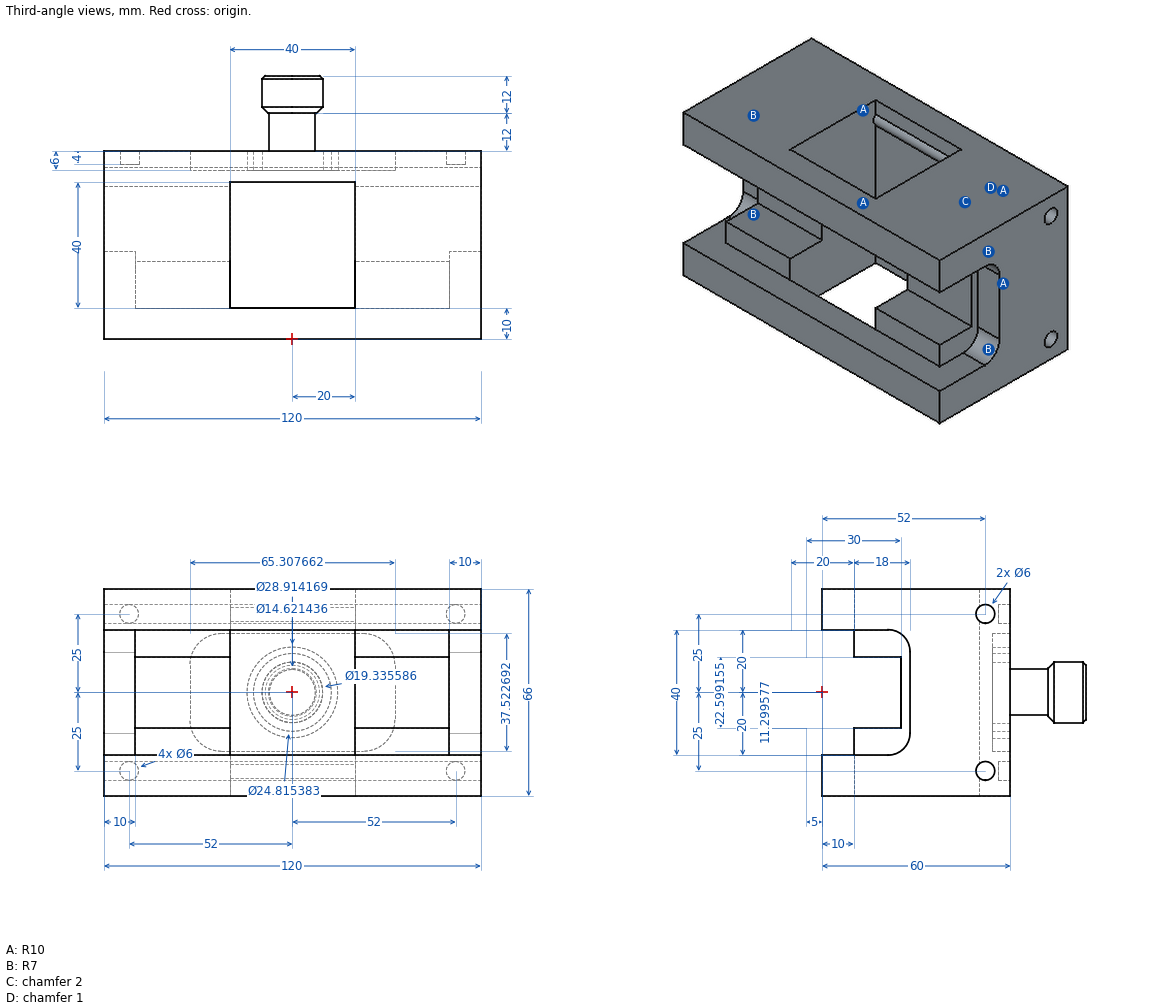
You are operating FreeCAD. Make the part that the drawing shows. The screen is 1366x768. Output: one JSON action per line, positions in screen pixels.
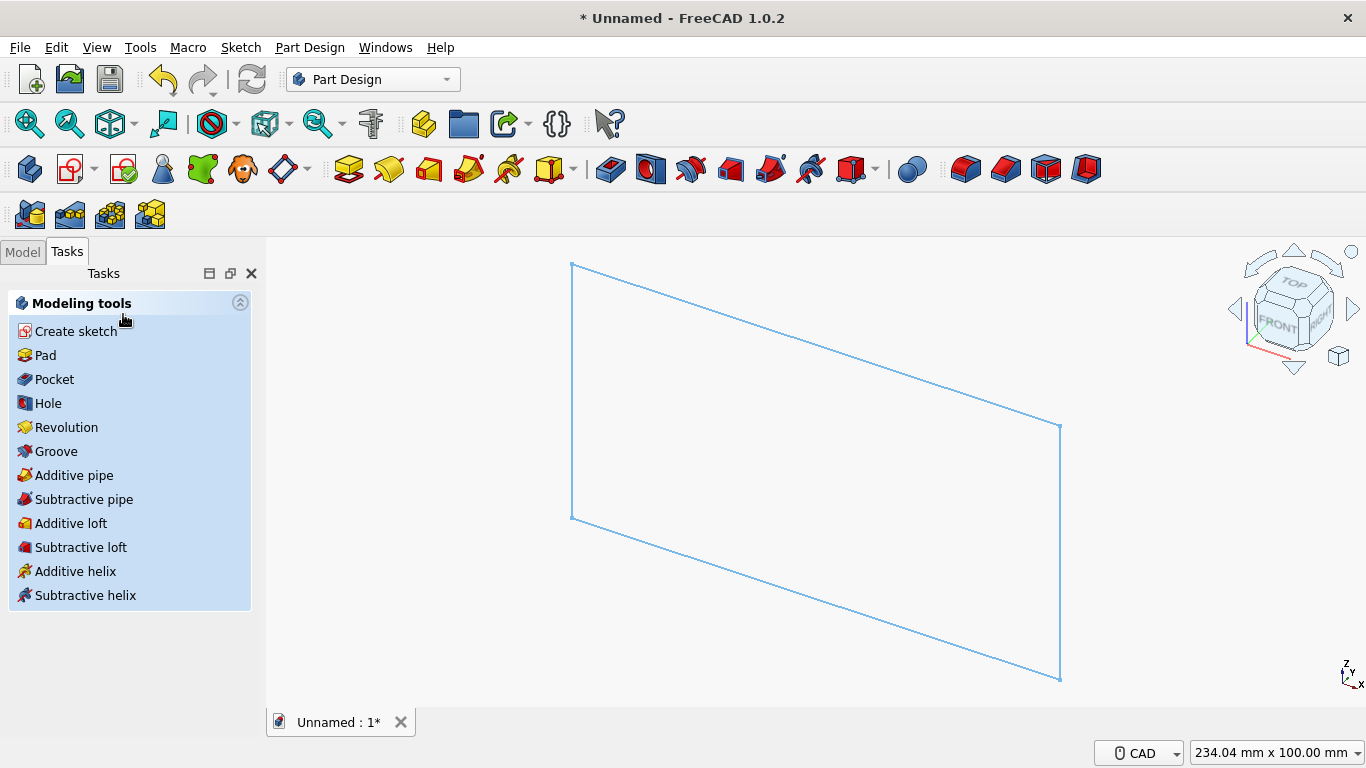
{"action": "left_click", "coordinate": [350, 170]}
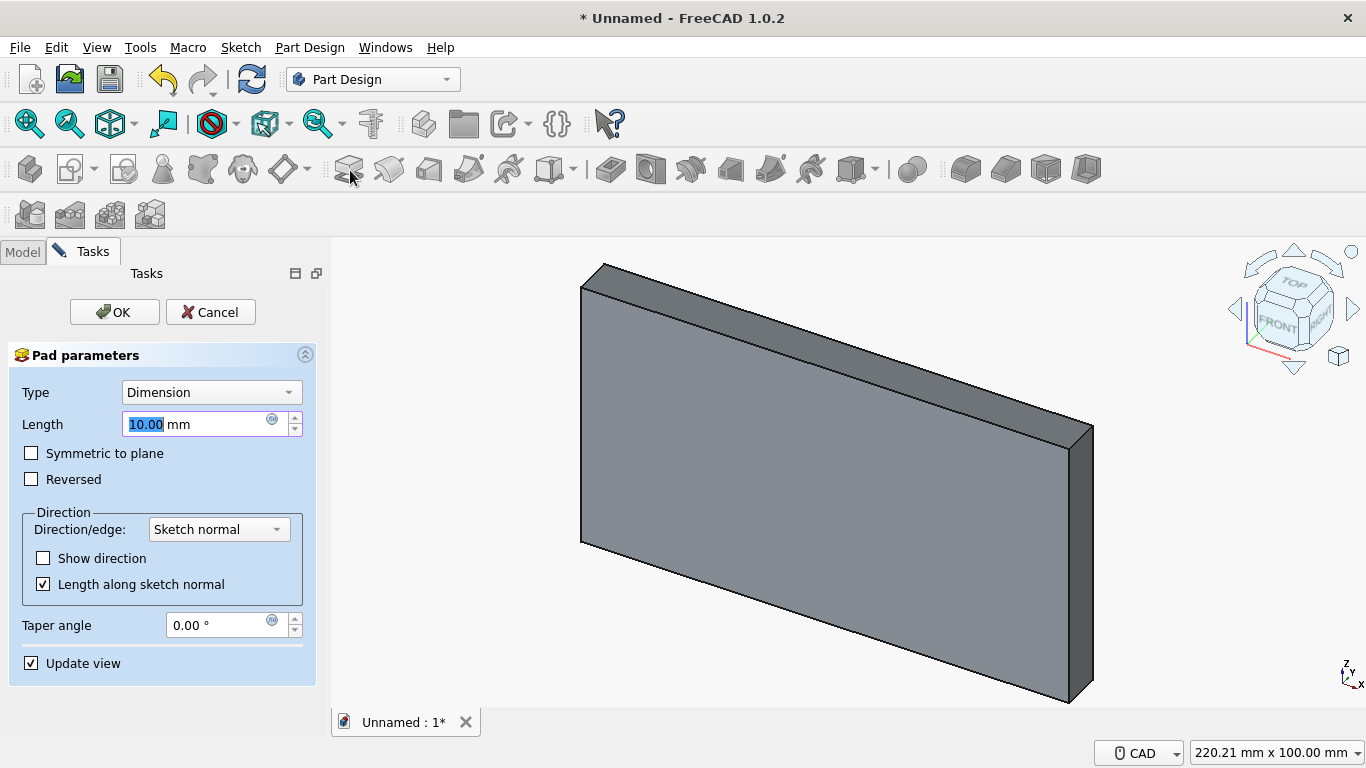
{"action": "type", "text": "60"}
{"action": "key", "text": "Tab"}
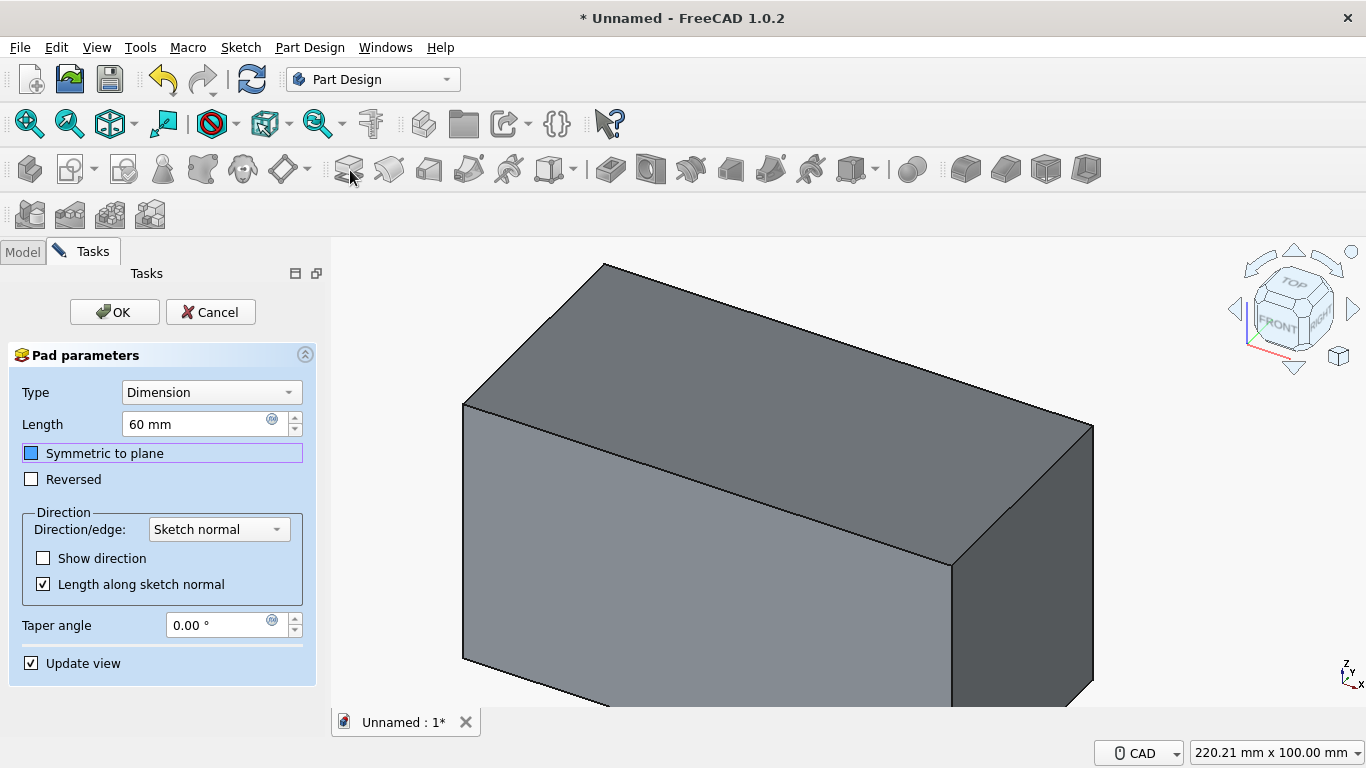
{"action": "left_click", "coordinate": [30, 479]}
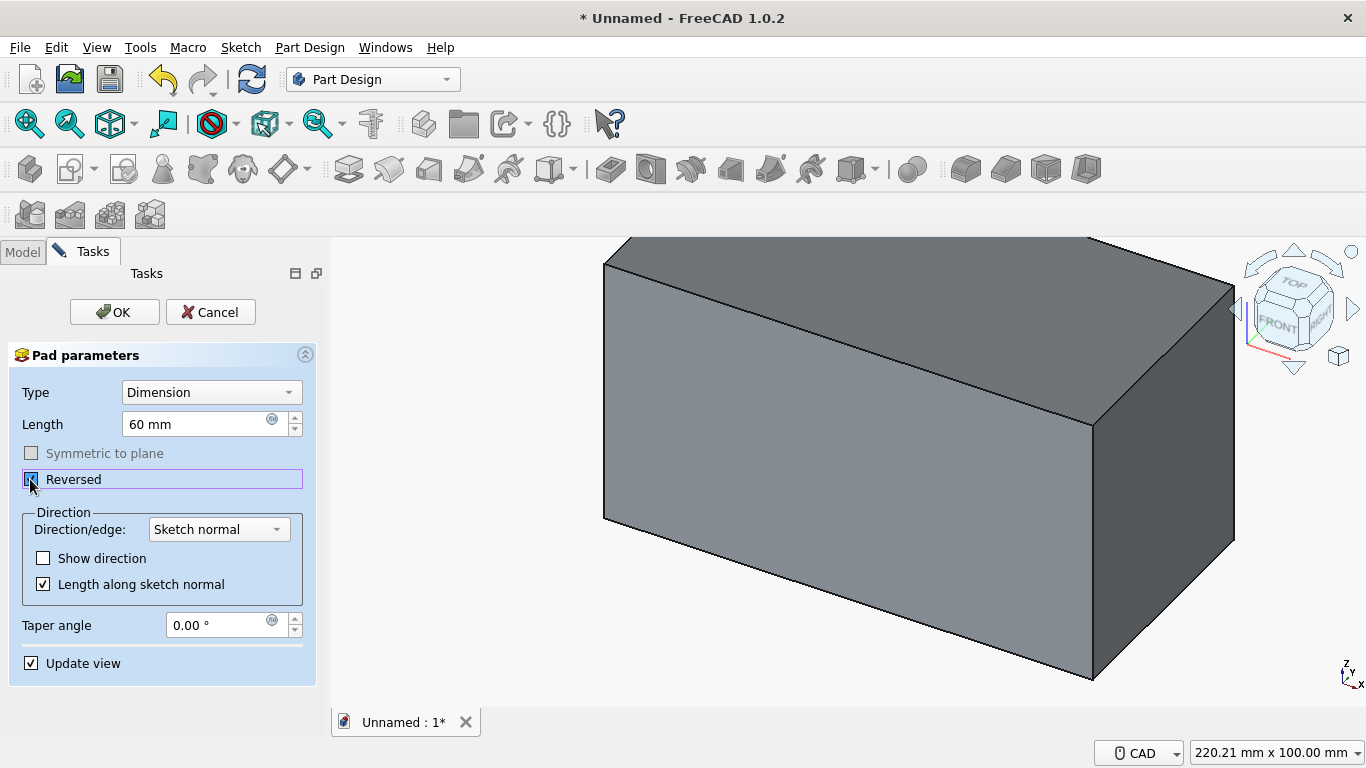
{"action": "left_click", "coordinate": [115, 312]}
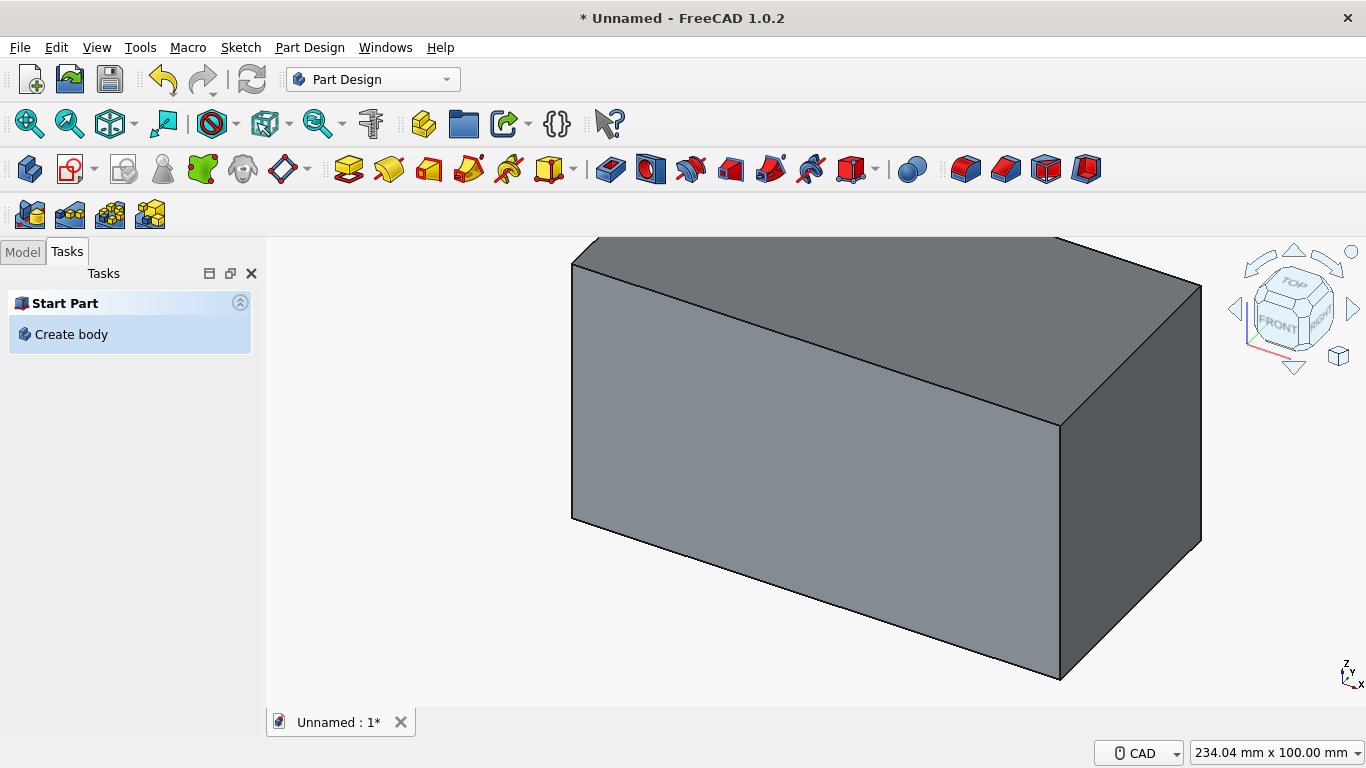
{"action": "left_click", "coordinate": [30, 124]}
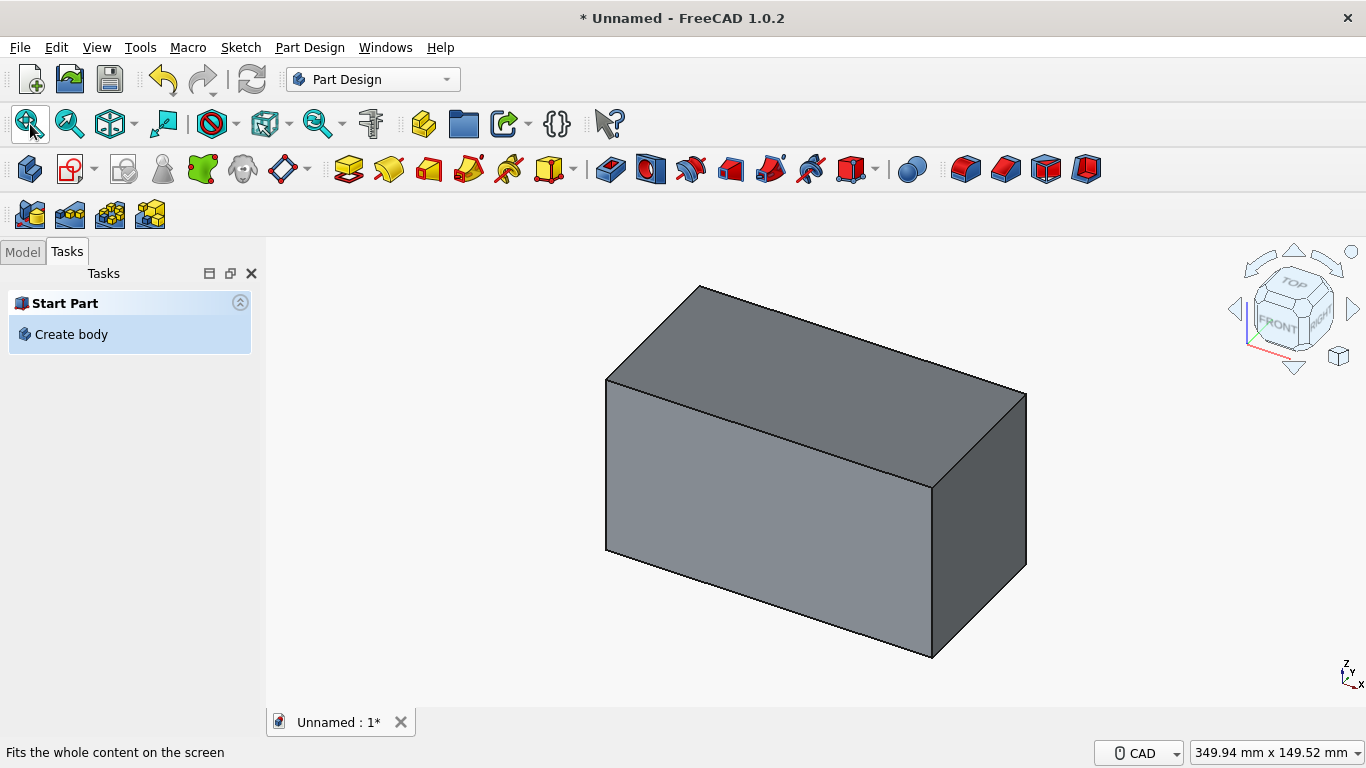
{"action": "left_click", "coordinate": [979, 525]}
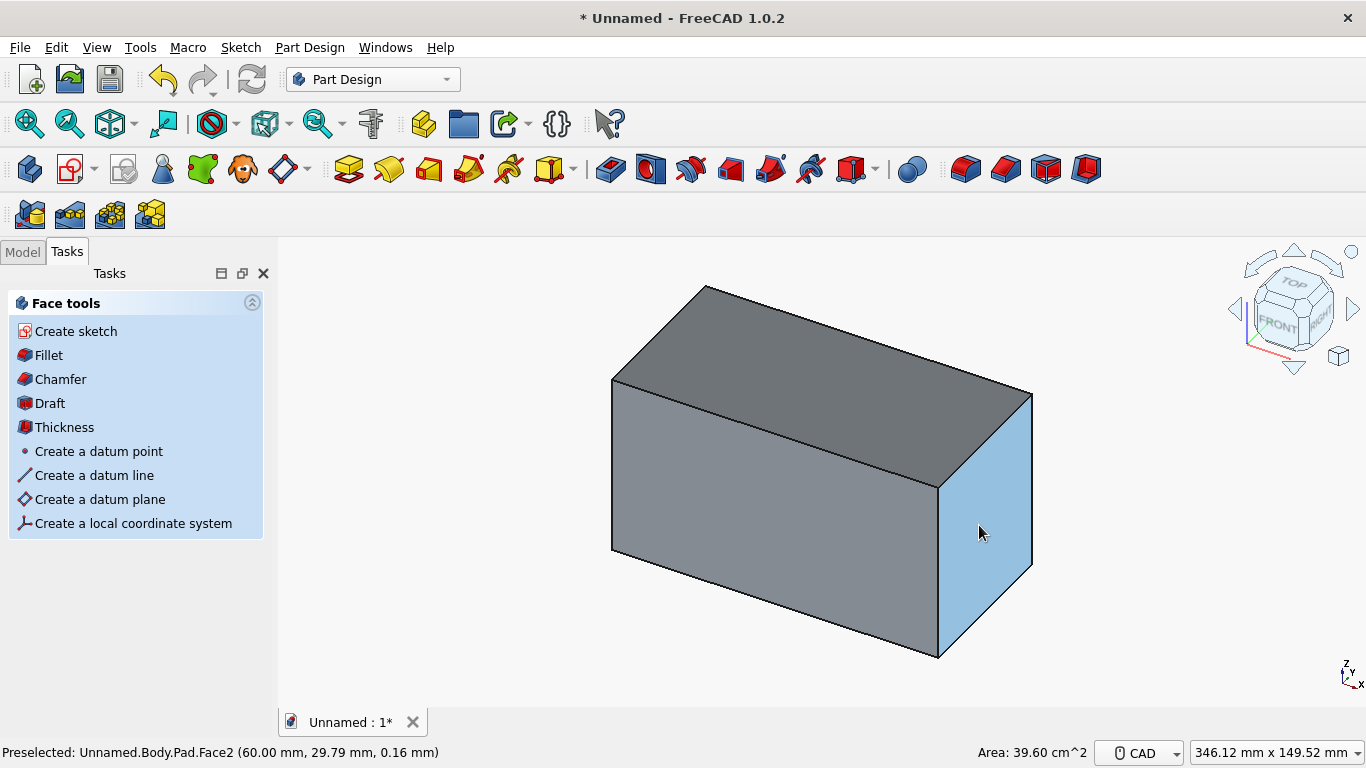
{"action": "left_click", "coordinate": [70, 170]}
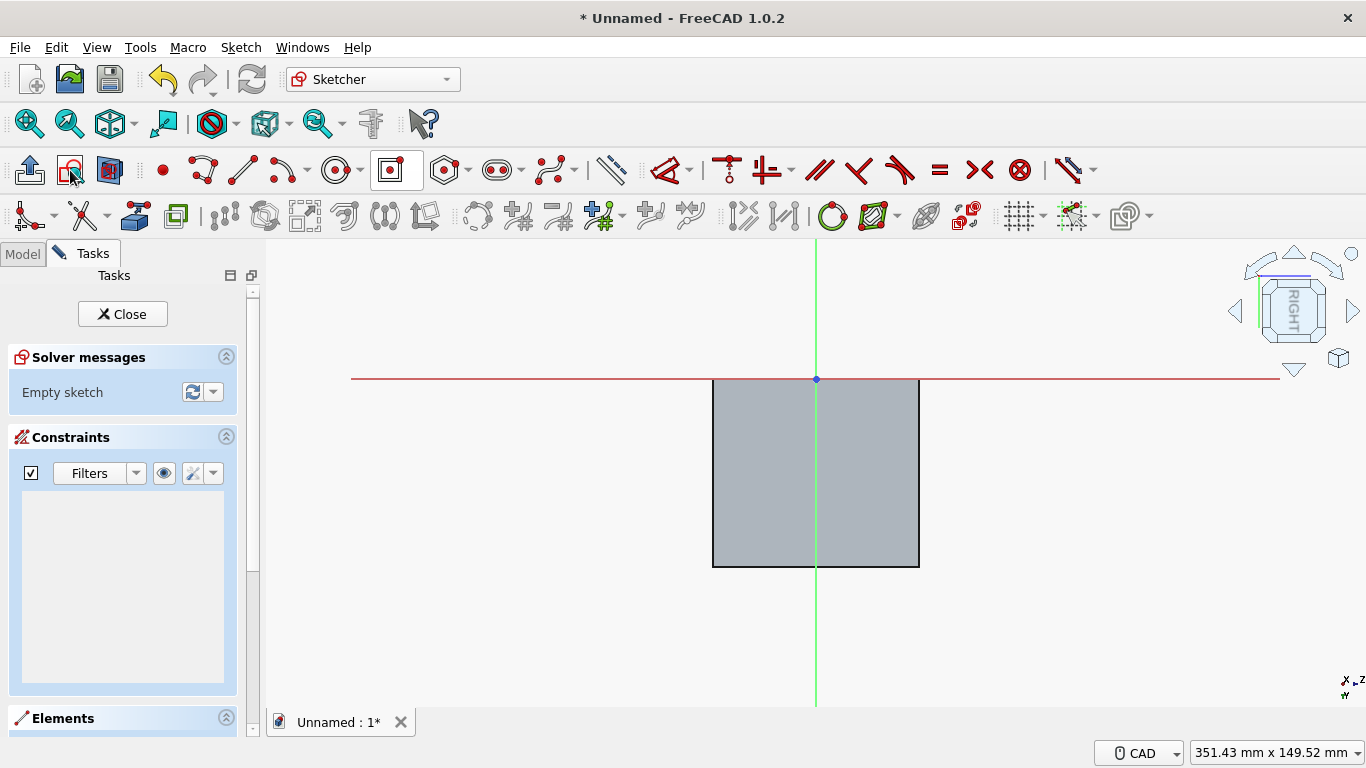
{"action": "scroll", "coordinate": [833, 355], "scroll_direction": "up", "scroll_amount": 8}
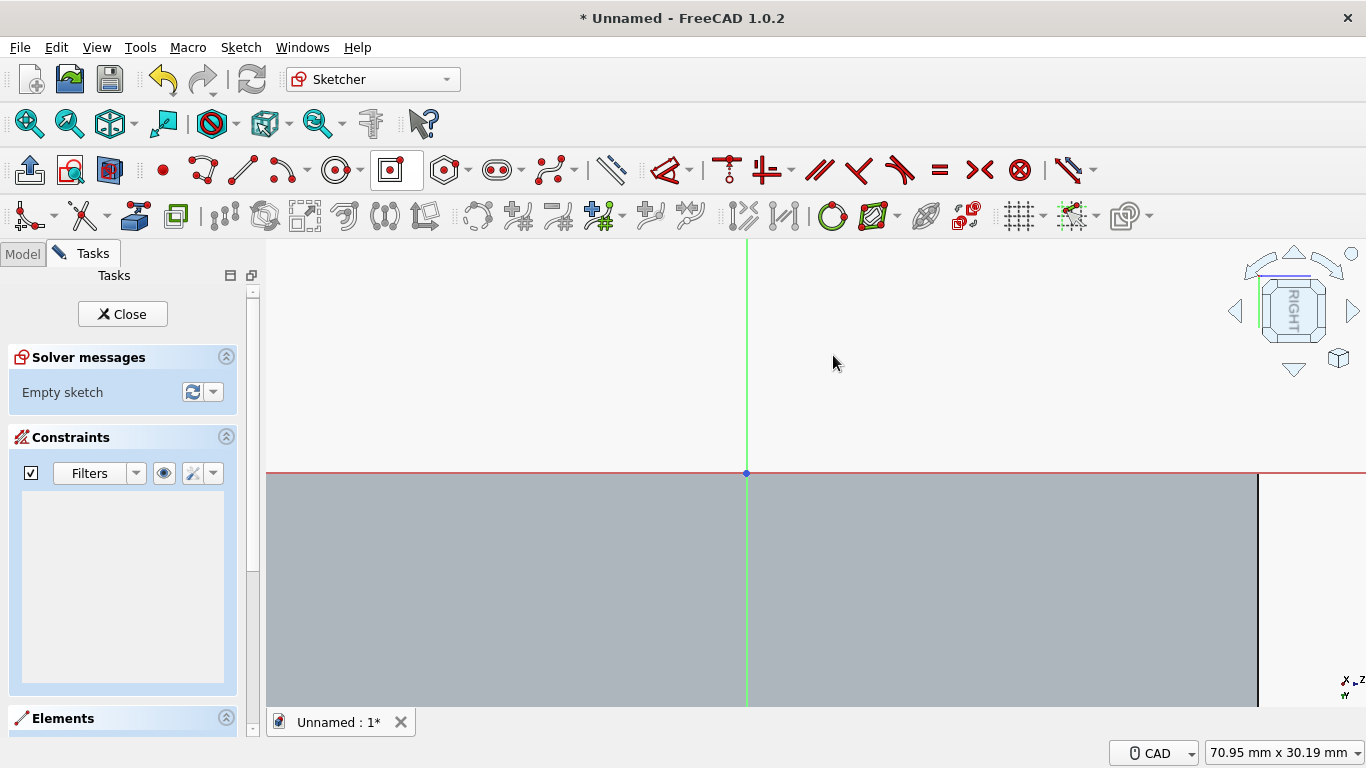
{"action": "left_click", "coordinate": [390, 170]}